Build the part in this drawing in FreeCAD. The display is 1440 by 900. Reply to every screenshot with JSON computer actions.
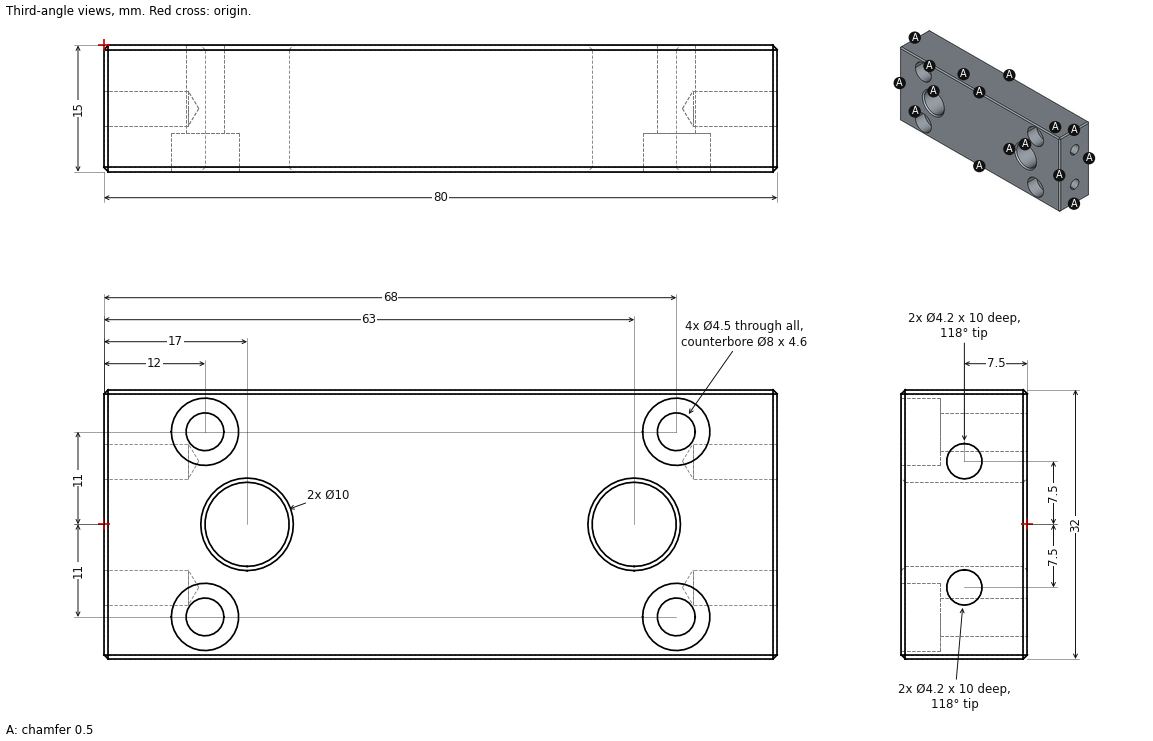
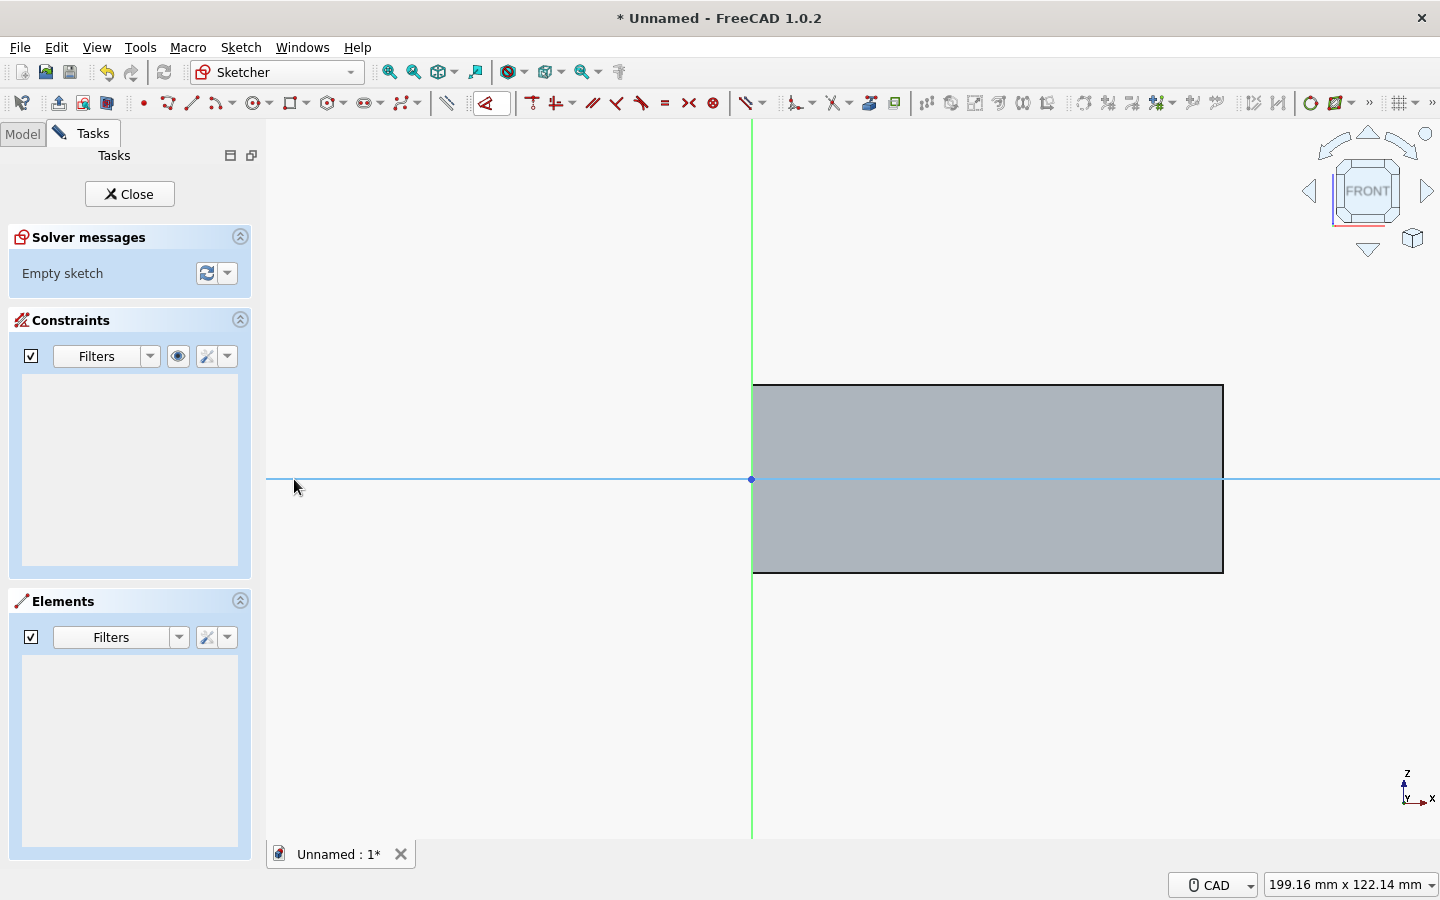
{"action": "scroll", "coordinate": [1171, 479], "scroll_direction": "up", "scroll_amount": 3}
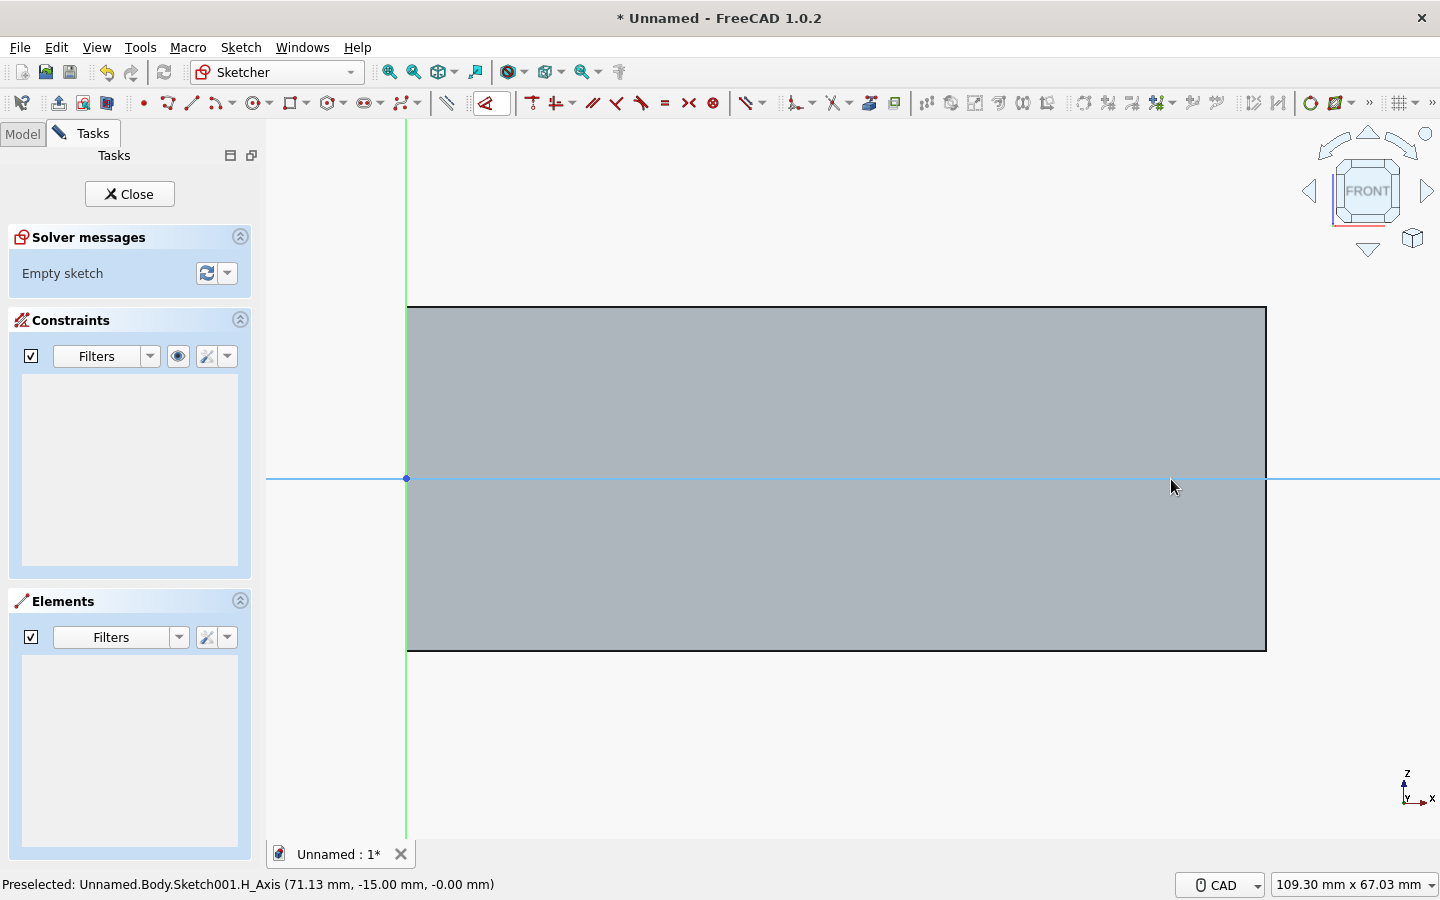
{"action": "left_click", "coordinate": [254, 104]}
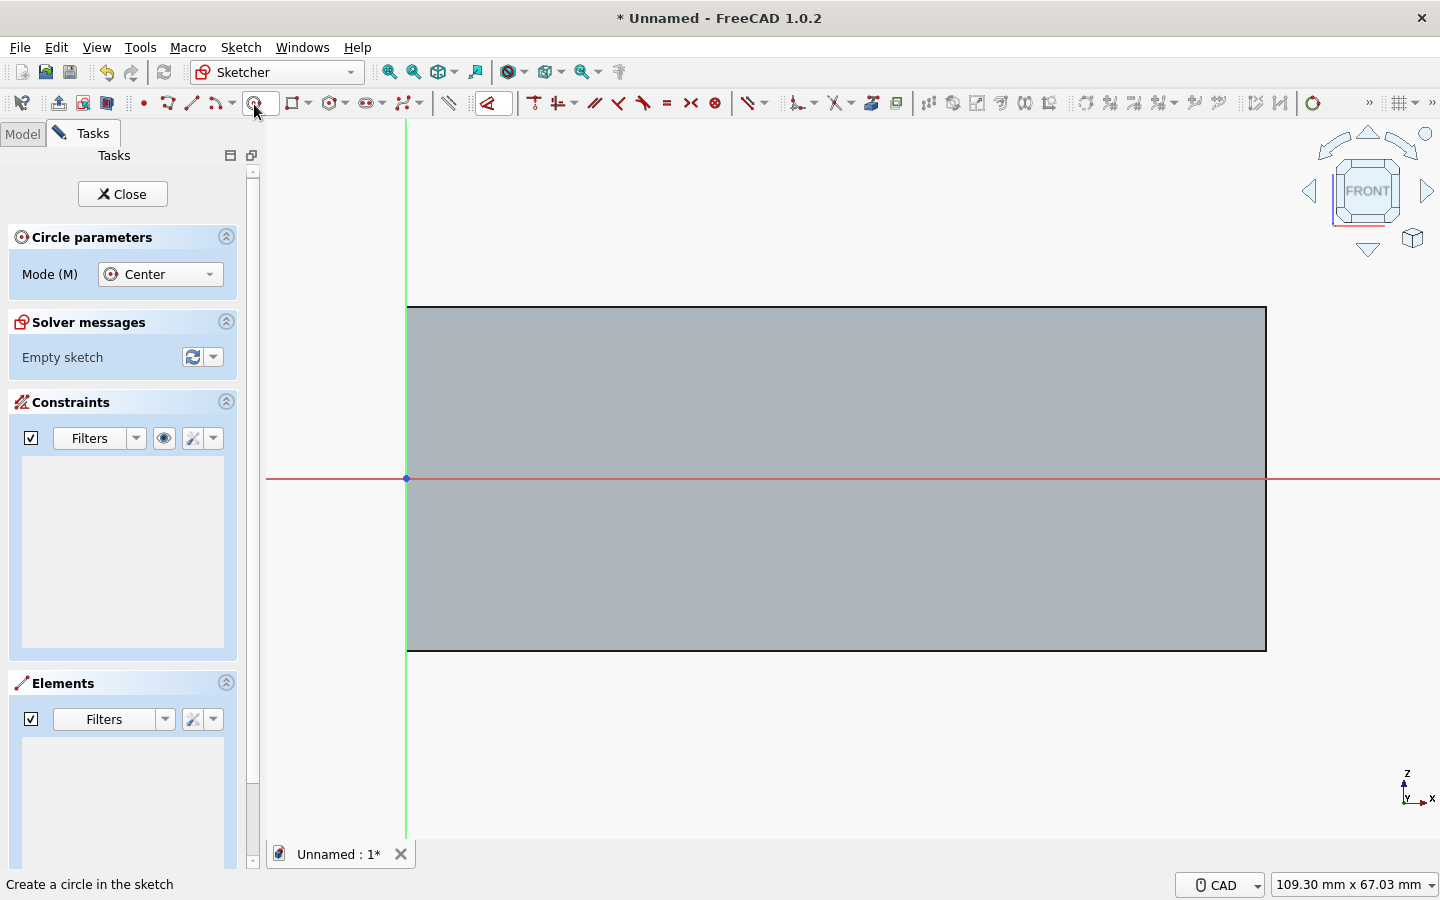
{"action": "left_click", "coordinate": [1137, 361]}
{"action": "left_click", "coordinate": [1154, 344]}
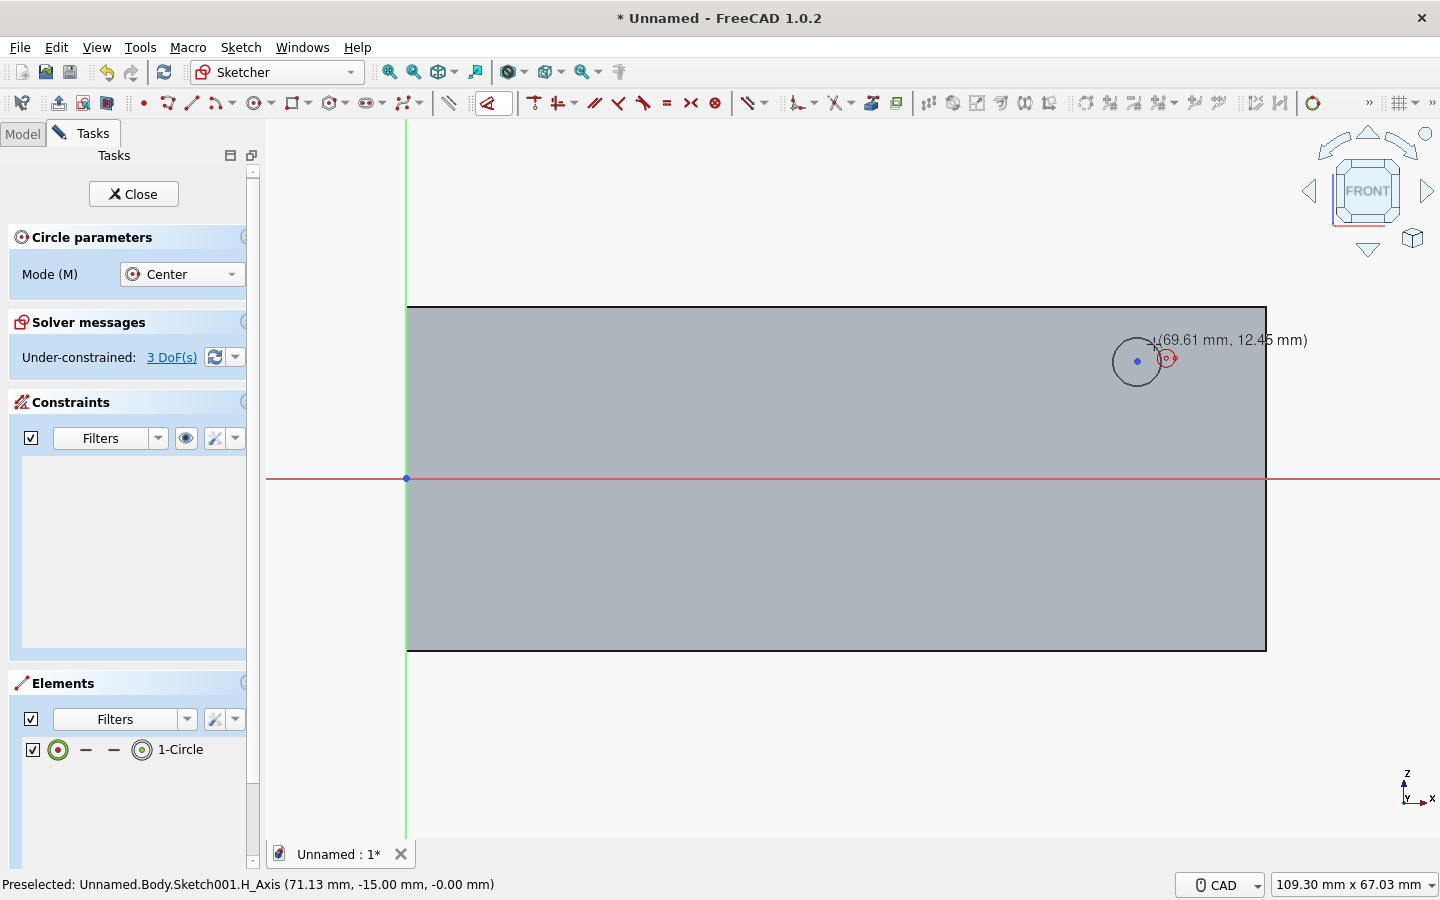
{"action": "left_click", "coordinate": [1137, 597]}
{"action": "left_click", "coordinate": [1154, 580]}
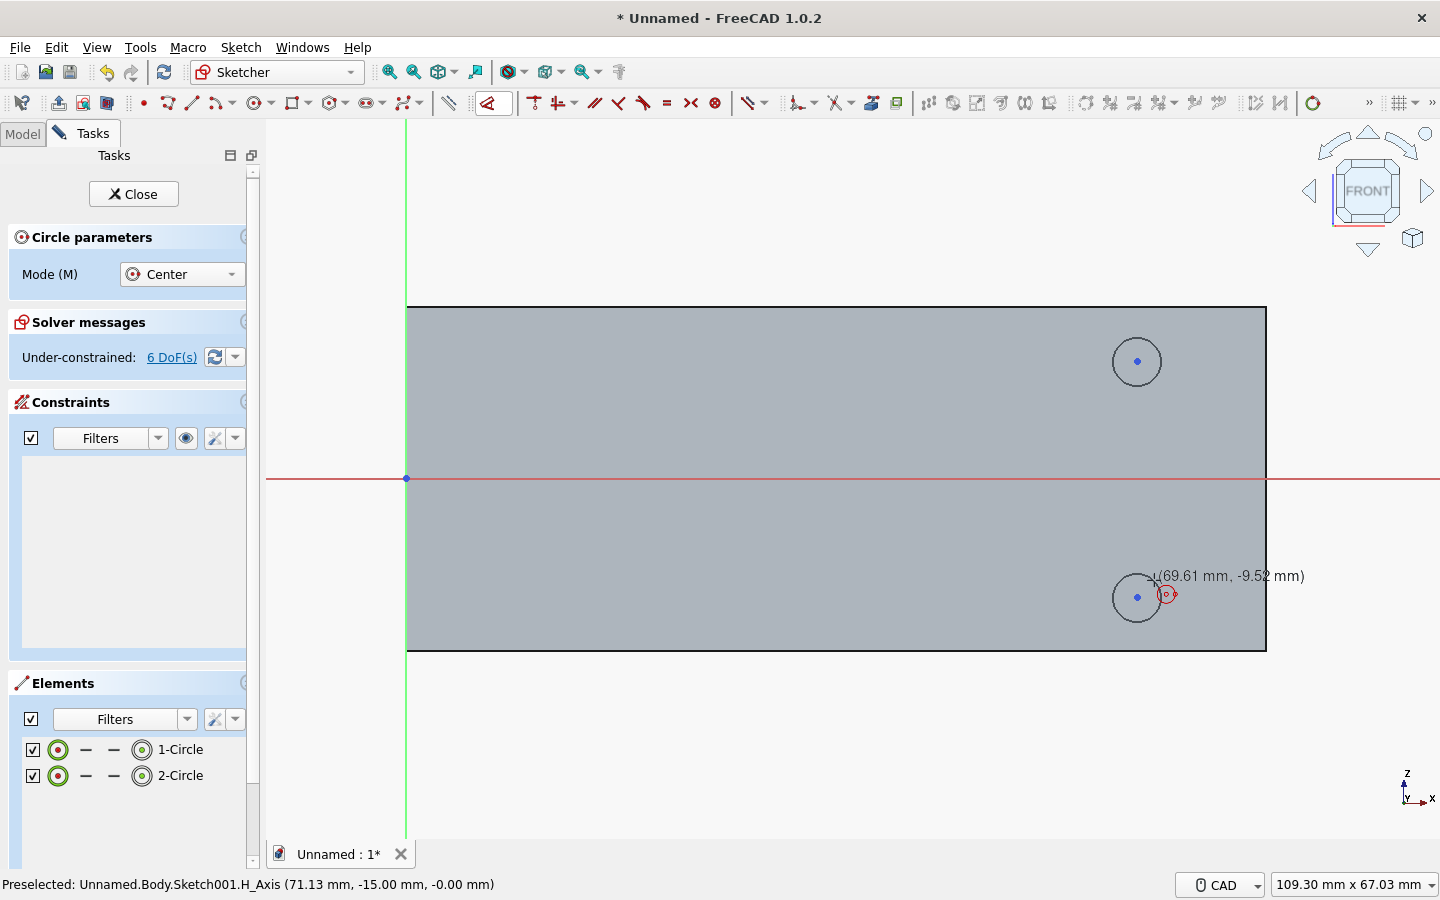
{"action": "left_click", "coordinate": [535, 361]}
{"action": "left_click", "coordinate": [552, 344]}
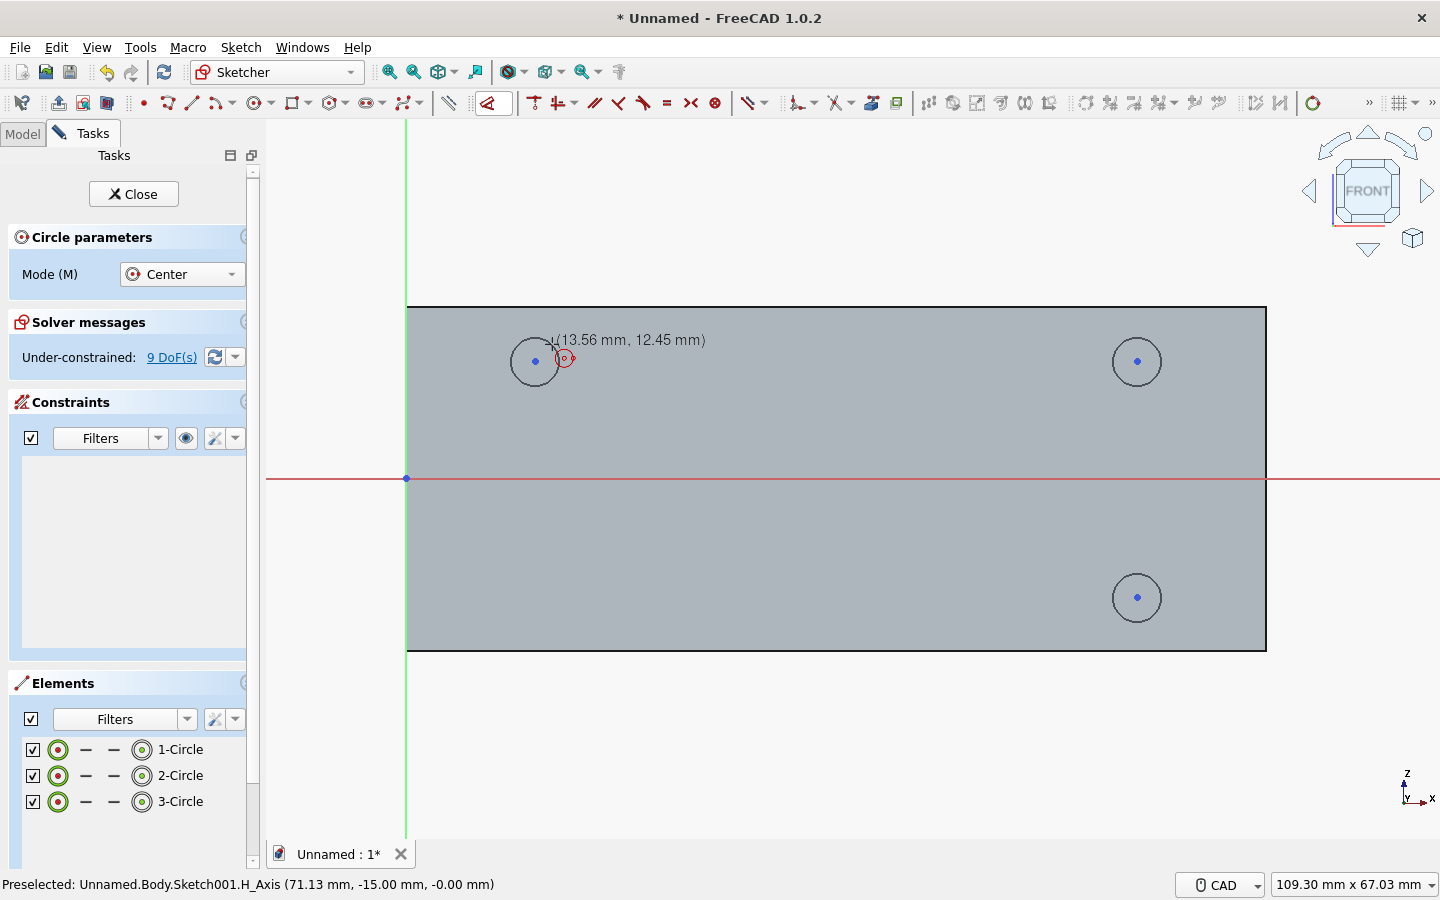
{"action": "left_click", "coordinate": [535, 597]}
{"action": "left_click", "coordinate": [552, 580]}
{"action": "key", "text": "Escape"}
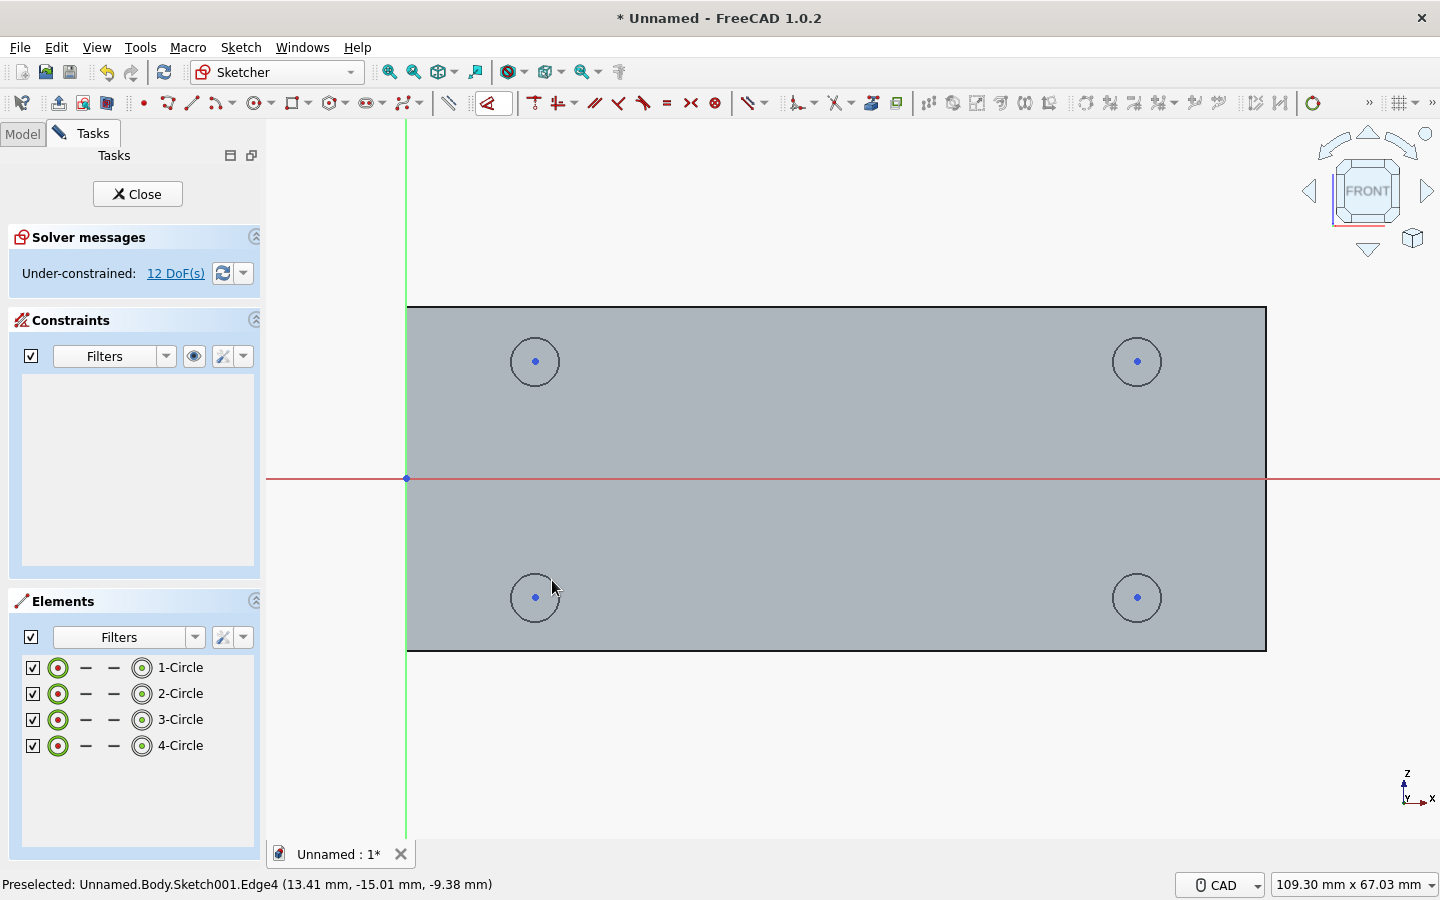
{"action": "left_click", "coordinate": [1154, 345]}